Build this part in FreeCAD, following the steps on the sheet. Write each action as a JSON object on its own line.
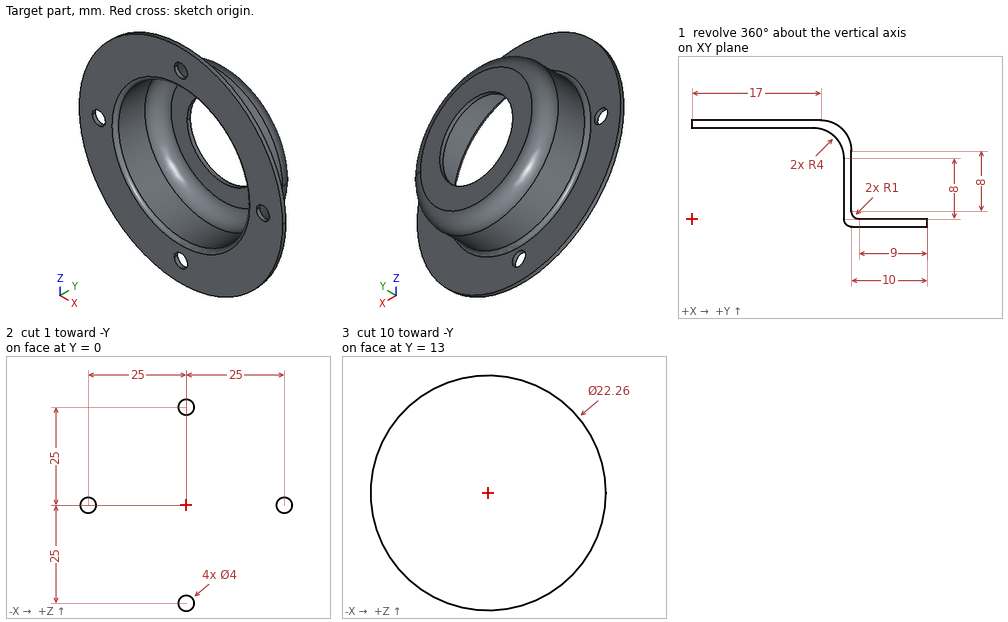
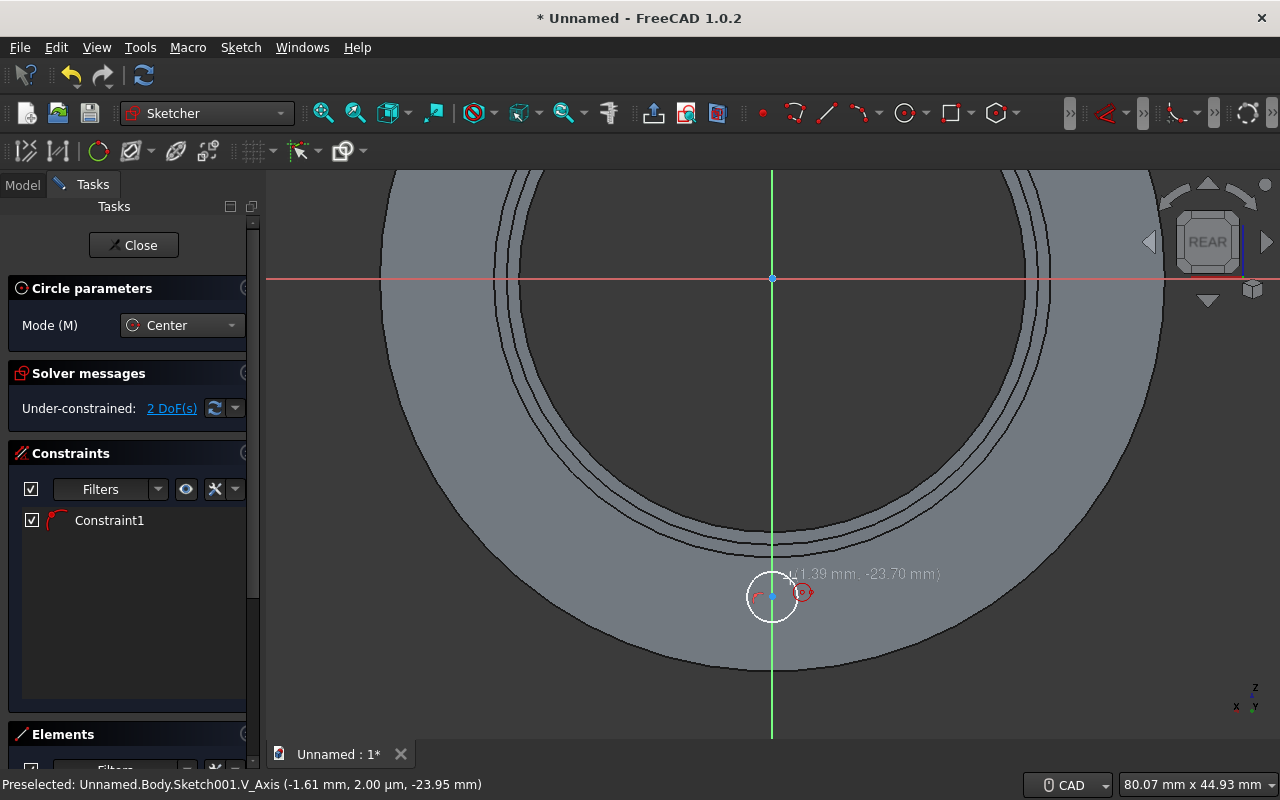
{"action": "left_click", "coordinate": [456, 279]}
{"action": "left_click", "coordinate": [474, 261]}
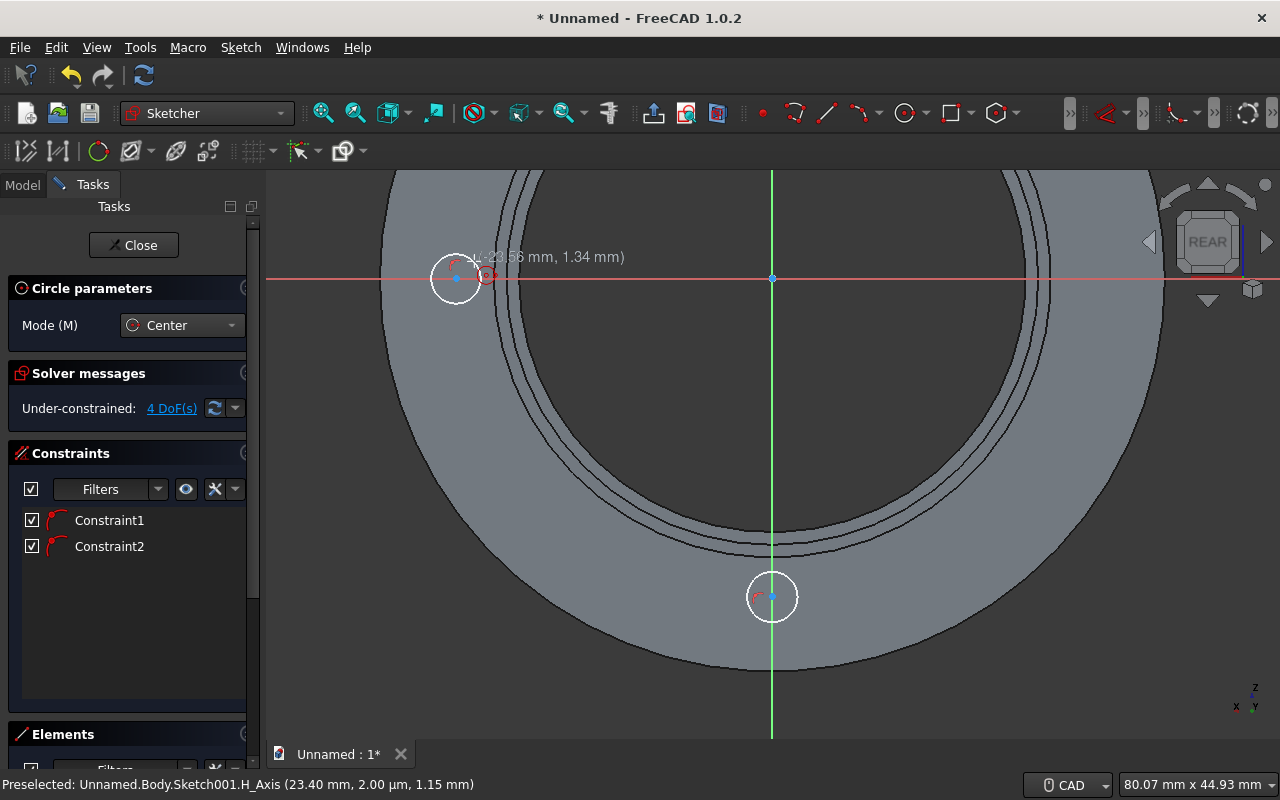
{"action": "scroll", "coordinate": [622, 668], "scroll_direction": "down", "scroll_amount": 3}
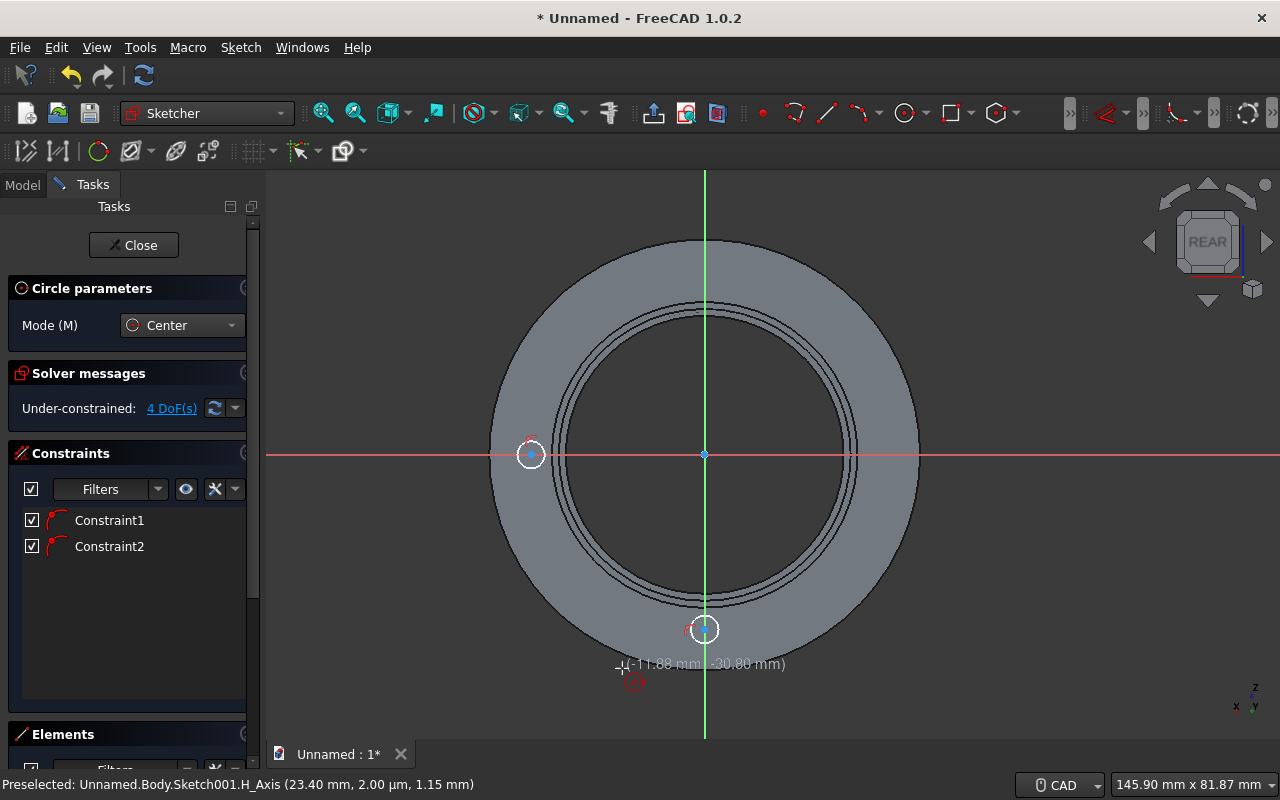
{"action": "scroll", "coordinate": [705, 281], "scroll_direction": "up", "scroll_amount": 3}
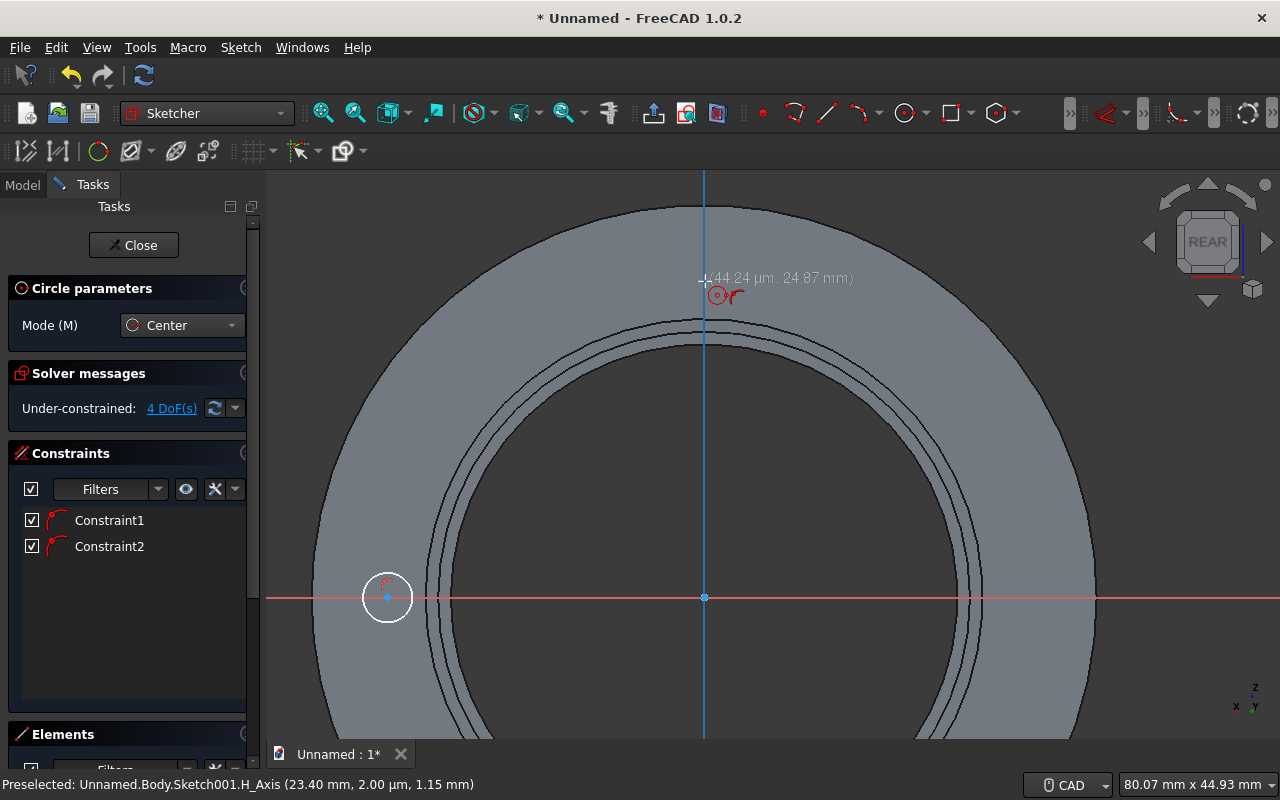
{"action": "left_click", "coordinate": [704, 281]}
{"action": "left_click", "coordinate": [722, 263]}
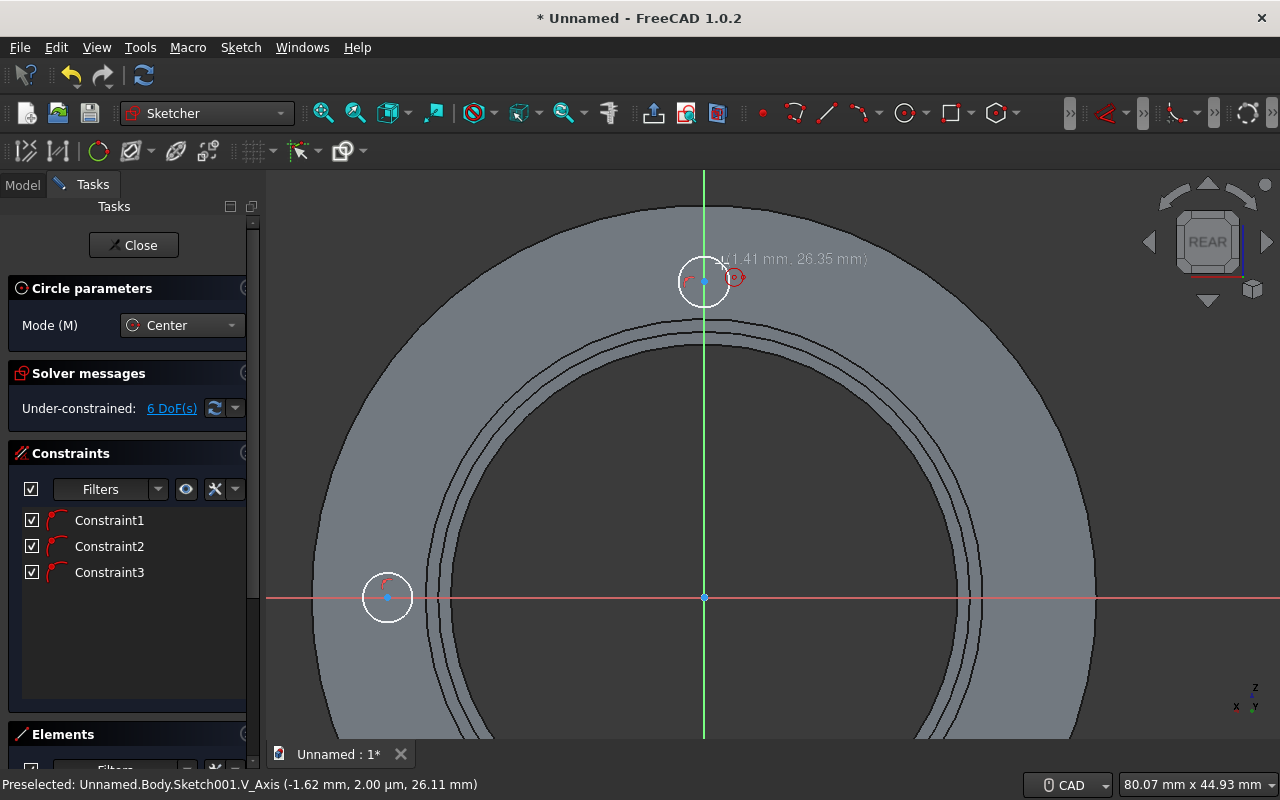
{"action": "left_click", "coordinate": [1021, 598]}
{"action": "left_click", "coordinate": [1039, 580]}
{"action": "key", "text": "Escape"}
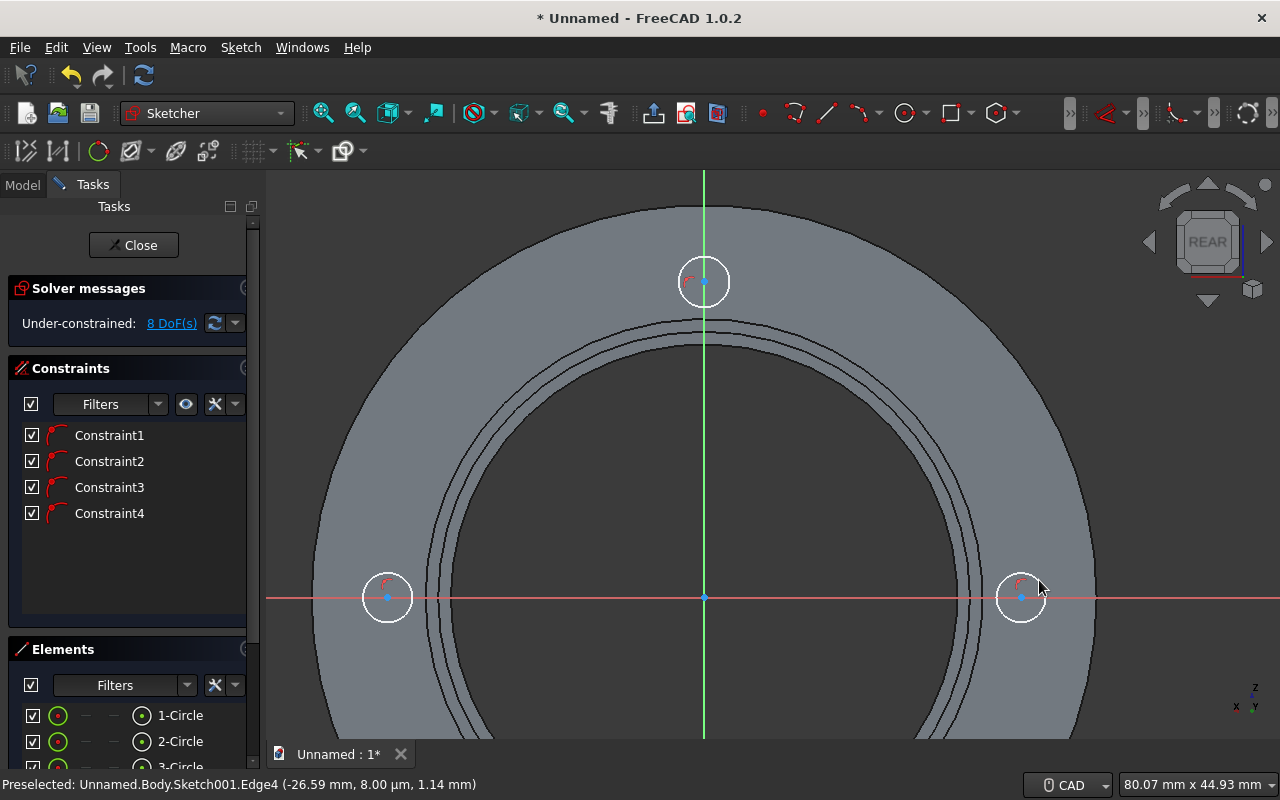
{"action": "scroll", "coordinate": [705, 280], "scroll_direction": "down", "scroll_amount": 3}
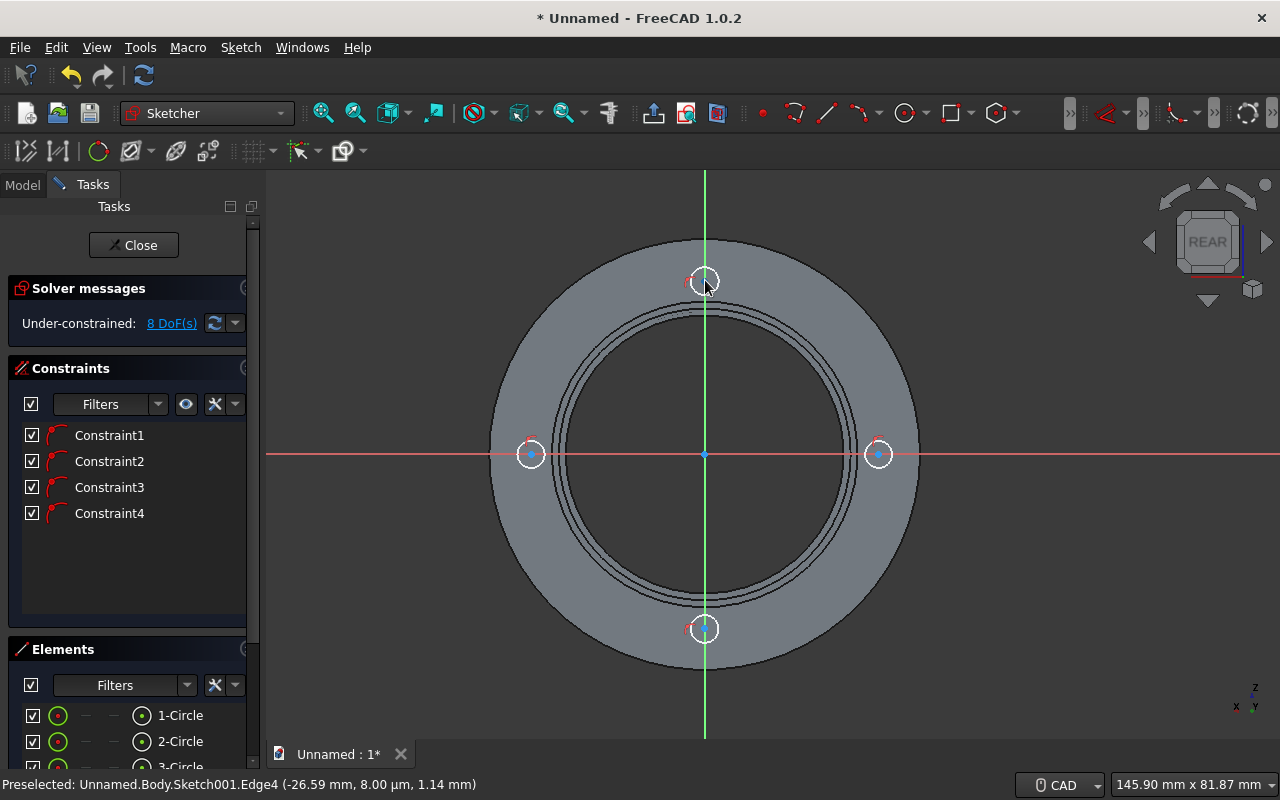
{"action": "scroll", "coordinate": [714, 619], "scroll_direction": "up", "scroll_amount": 2}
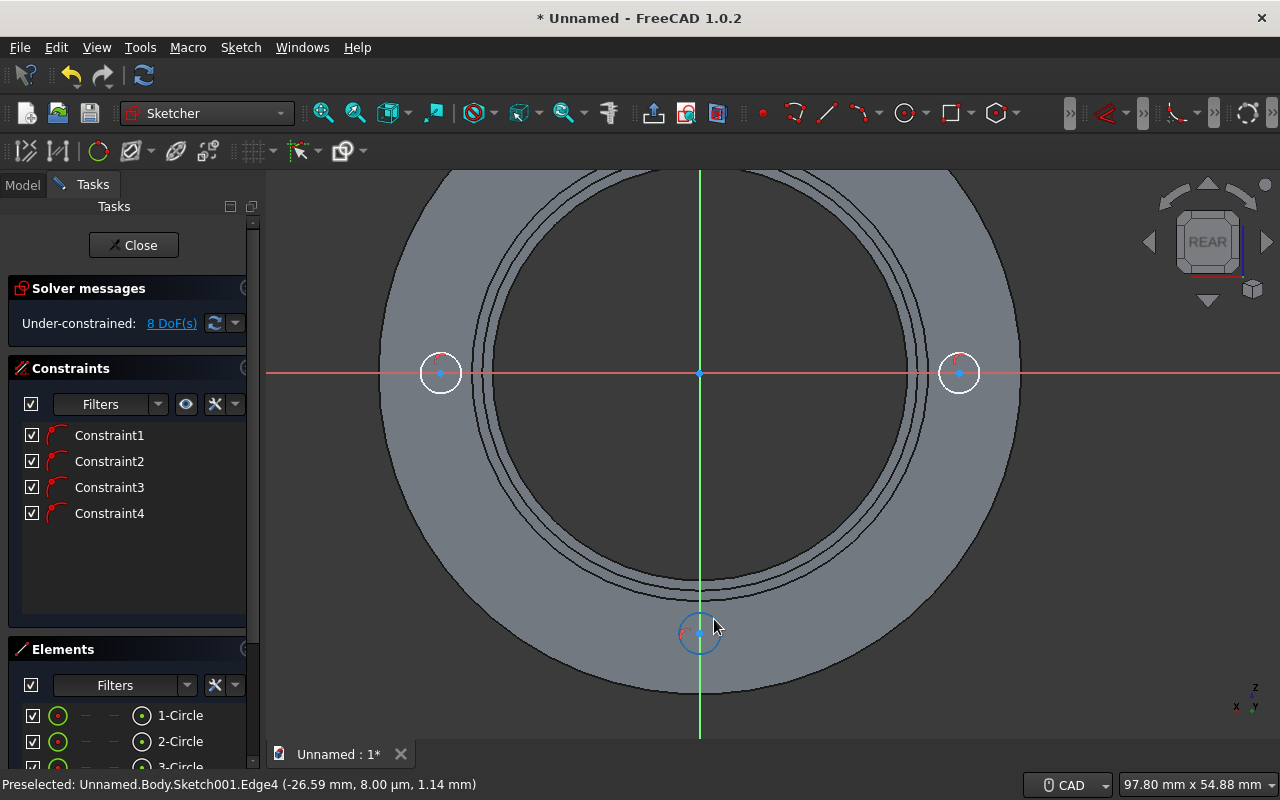
{"action": "left_click", "coordinate": [714, 619]}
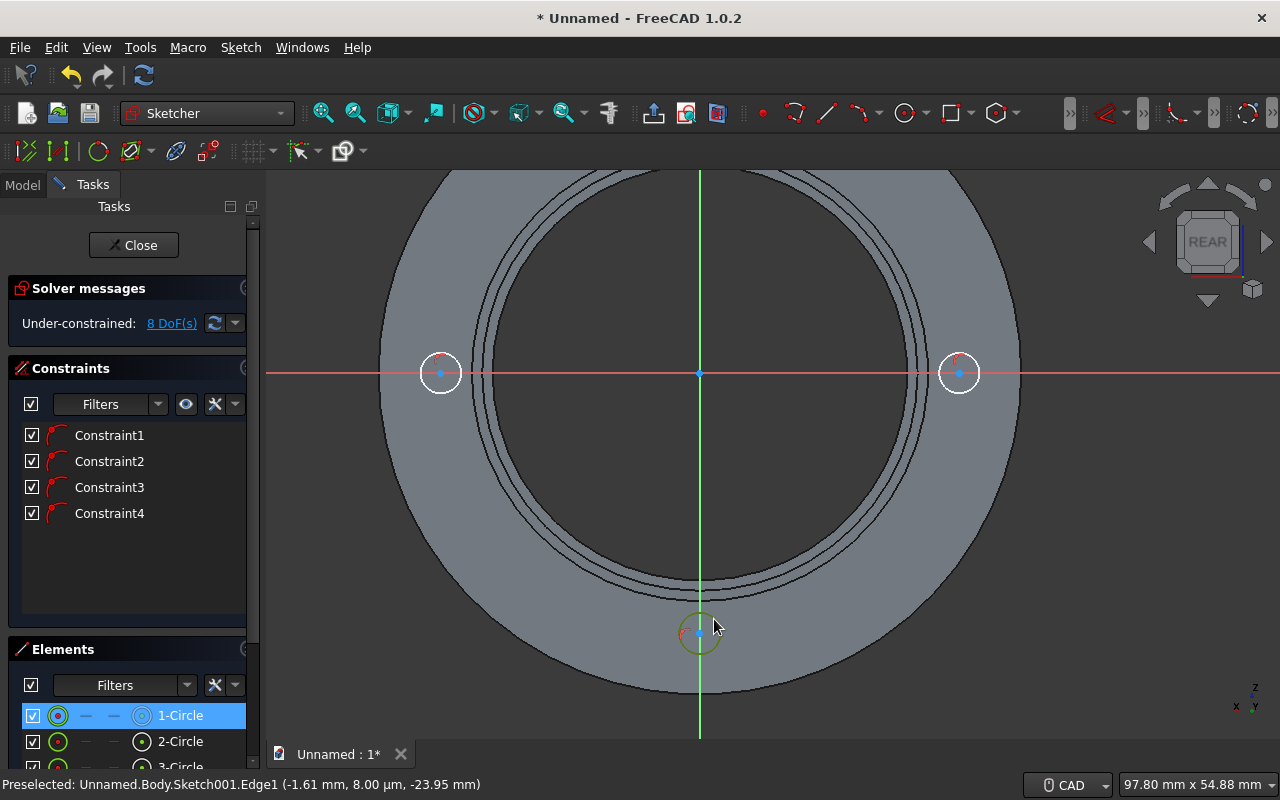
{"action": "left_click", "coordinate": [455, 359]}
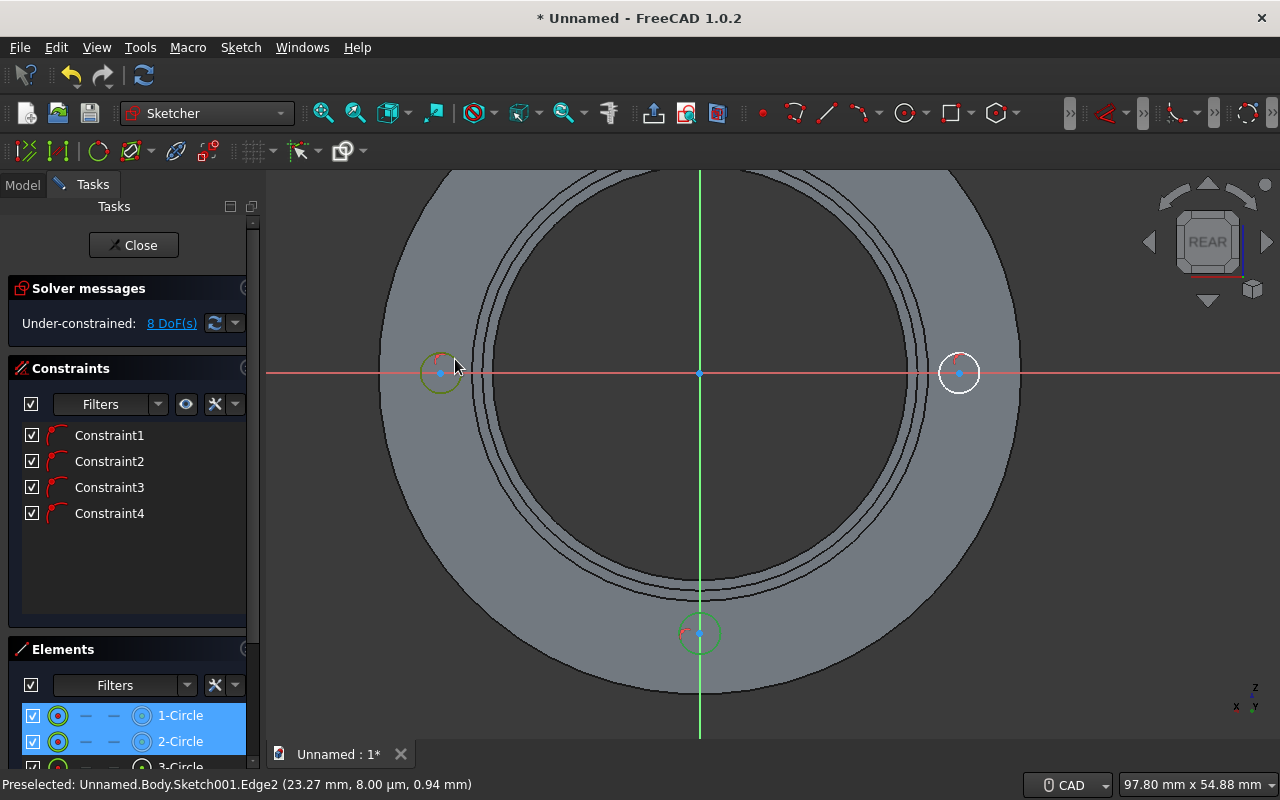
{"action": "scroll", "coordinate": [714, 620], "scroll_direction": "down", "scroll_amount": 2}